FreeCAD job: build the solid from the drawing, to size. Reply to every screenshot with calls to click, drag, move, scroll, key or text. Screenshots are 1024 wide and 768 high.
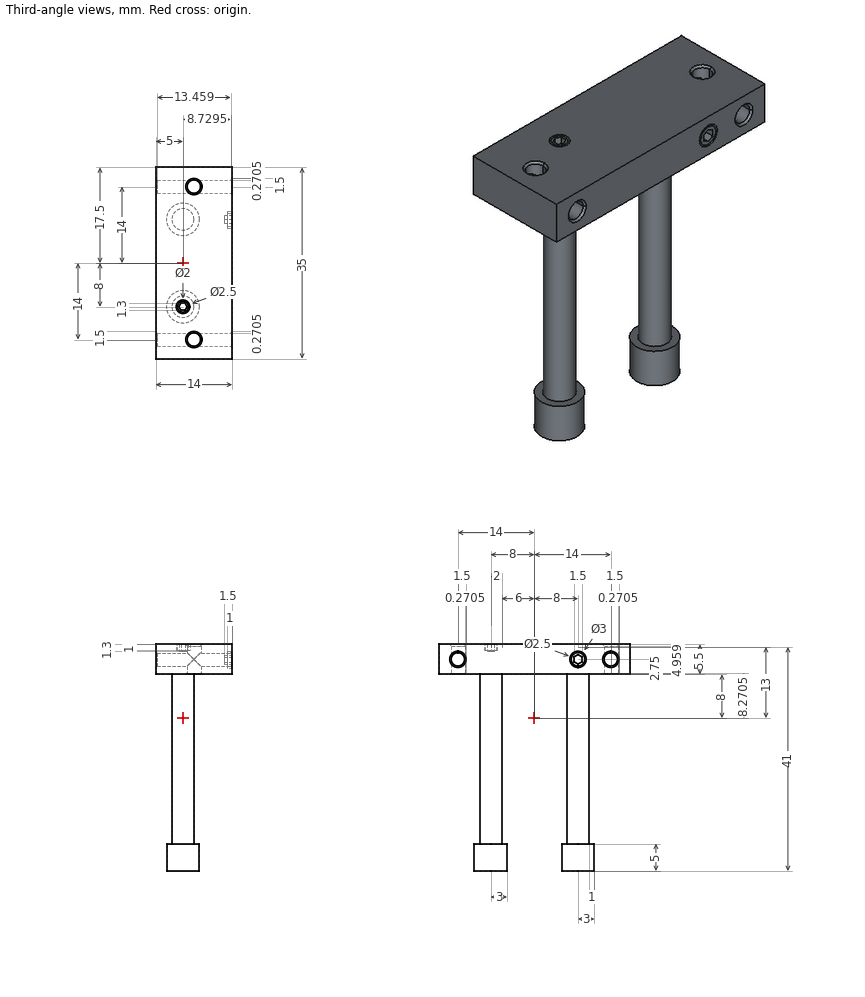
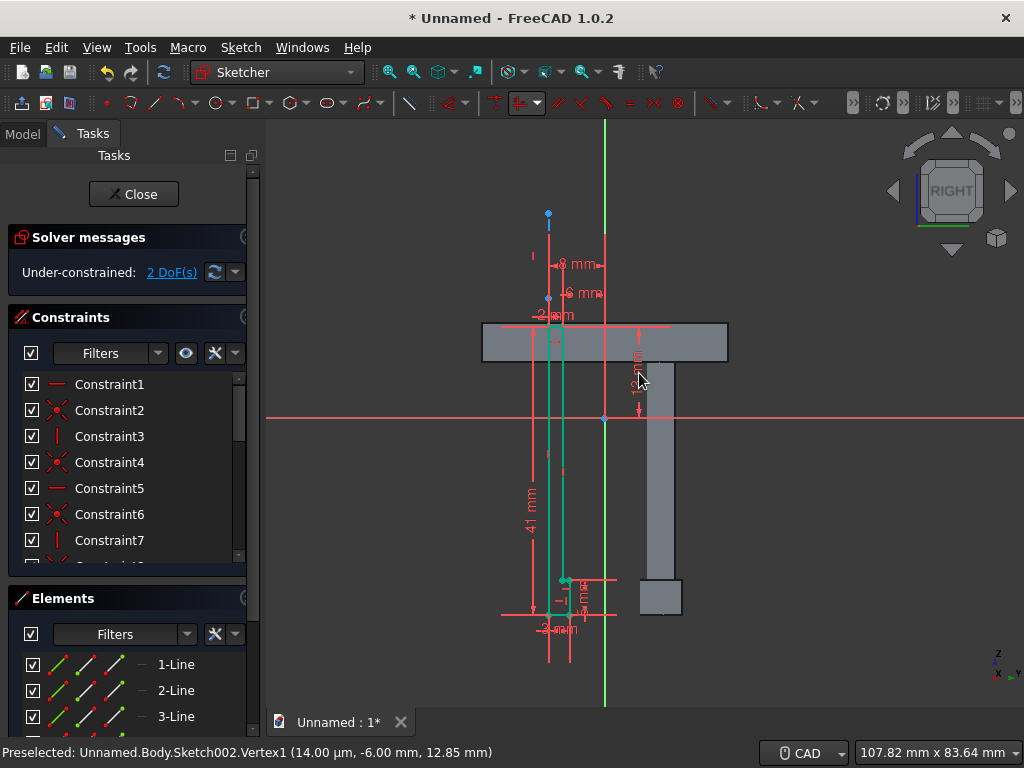
click(134, 194)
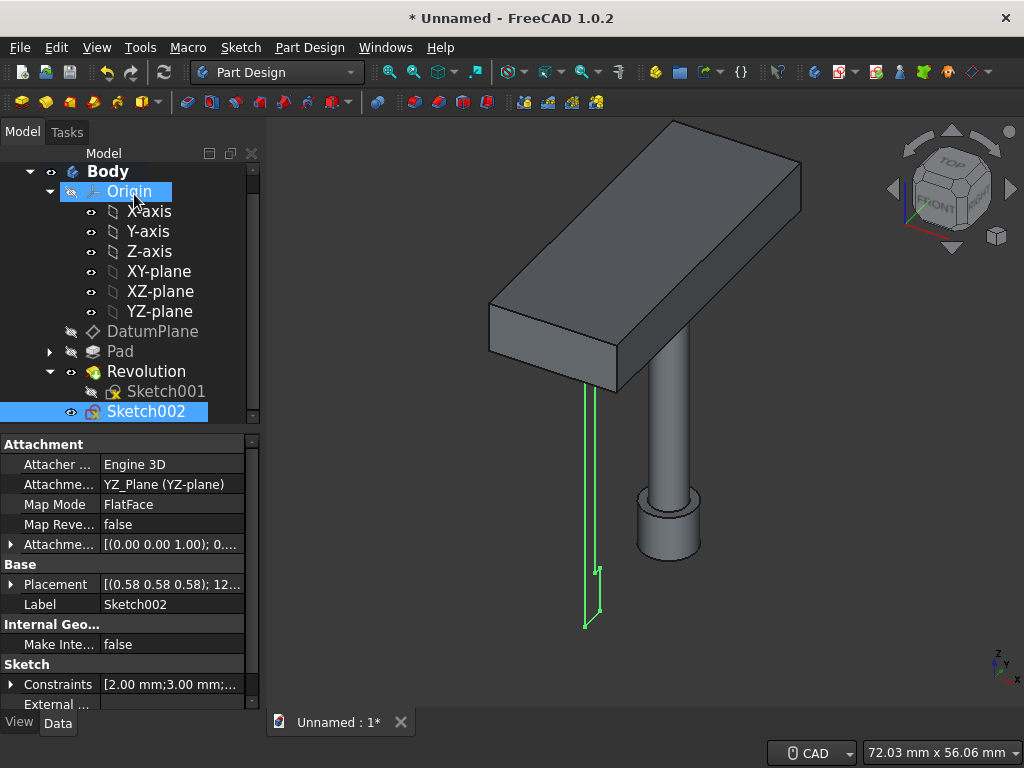
click(46, 102)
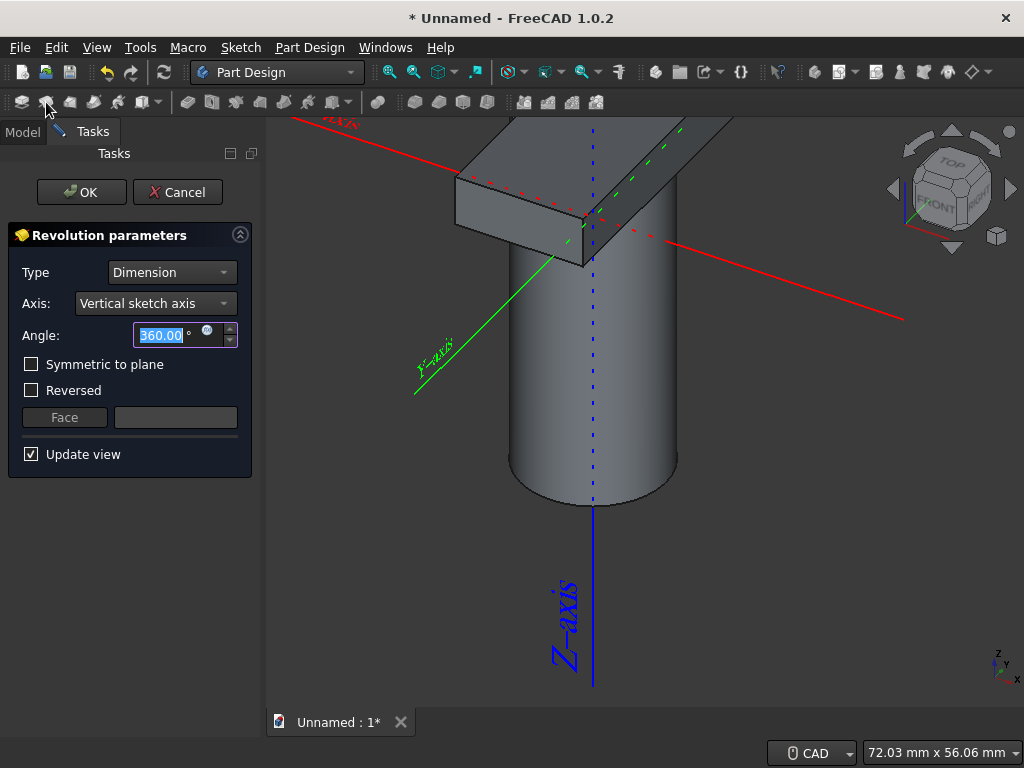
click(156, 304)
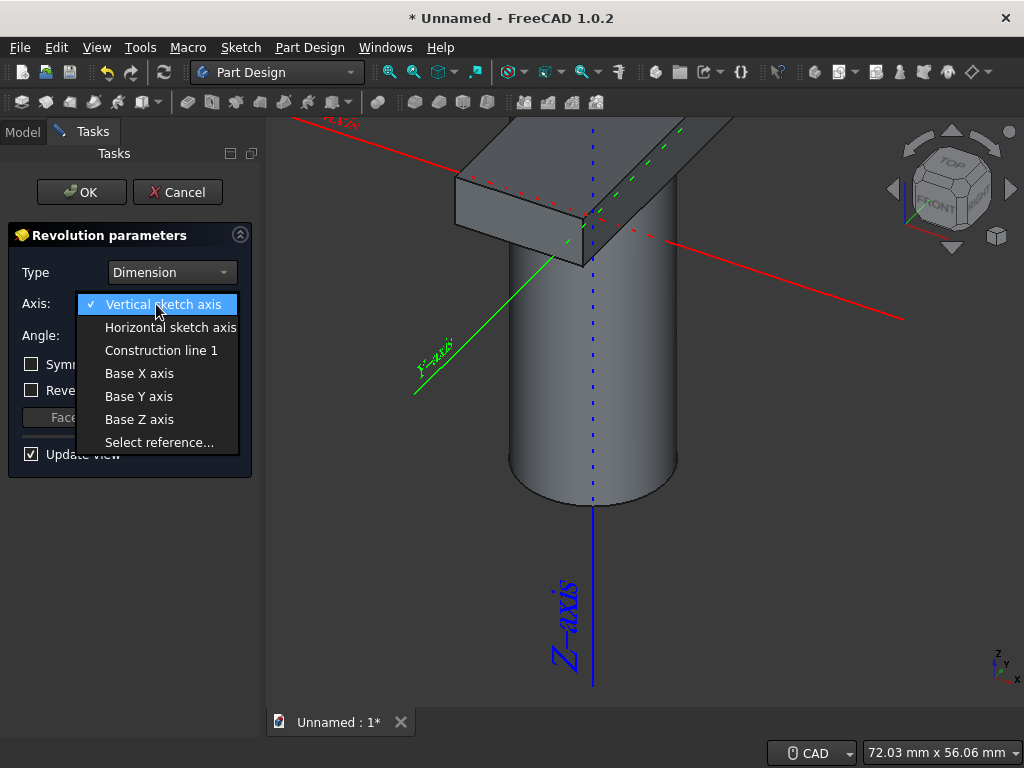
click(156, 350)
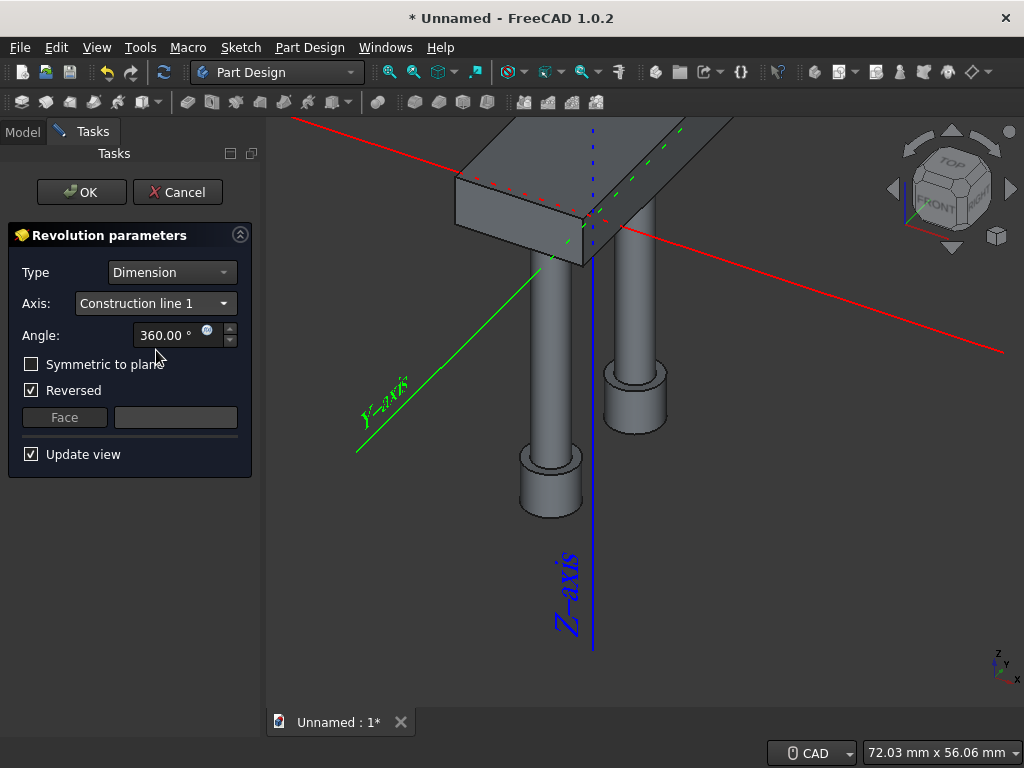
click(82, 192)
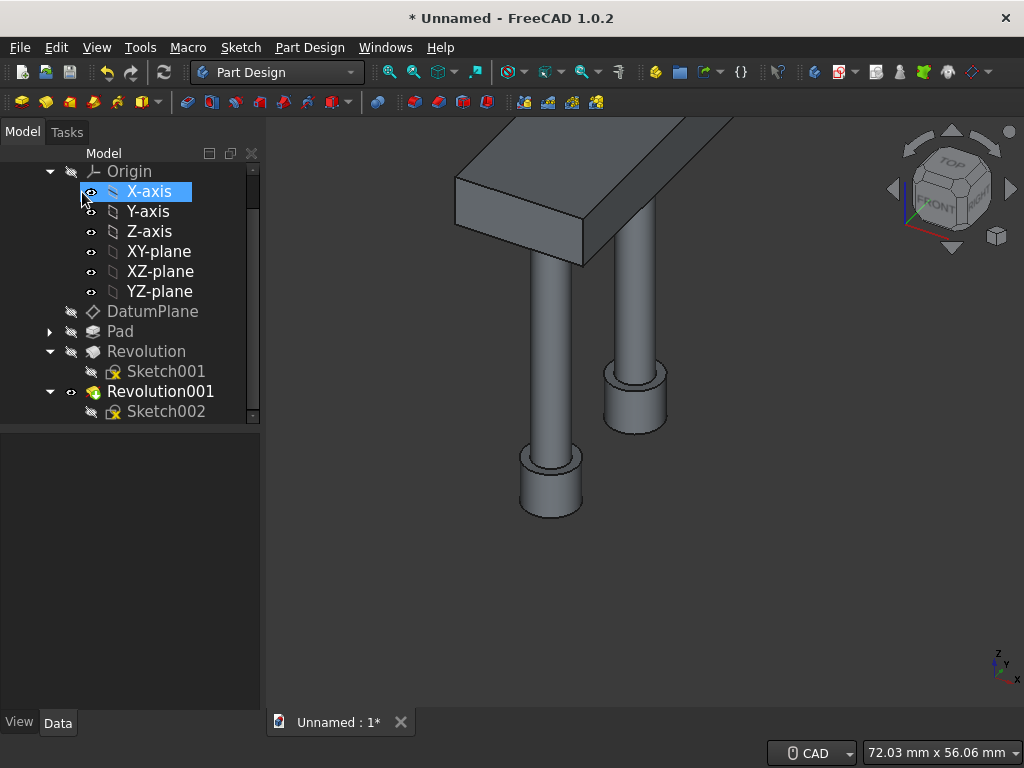
click(390, 72)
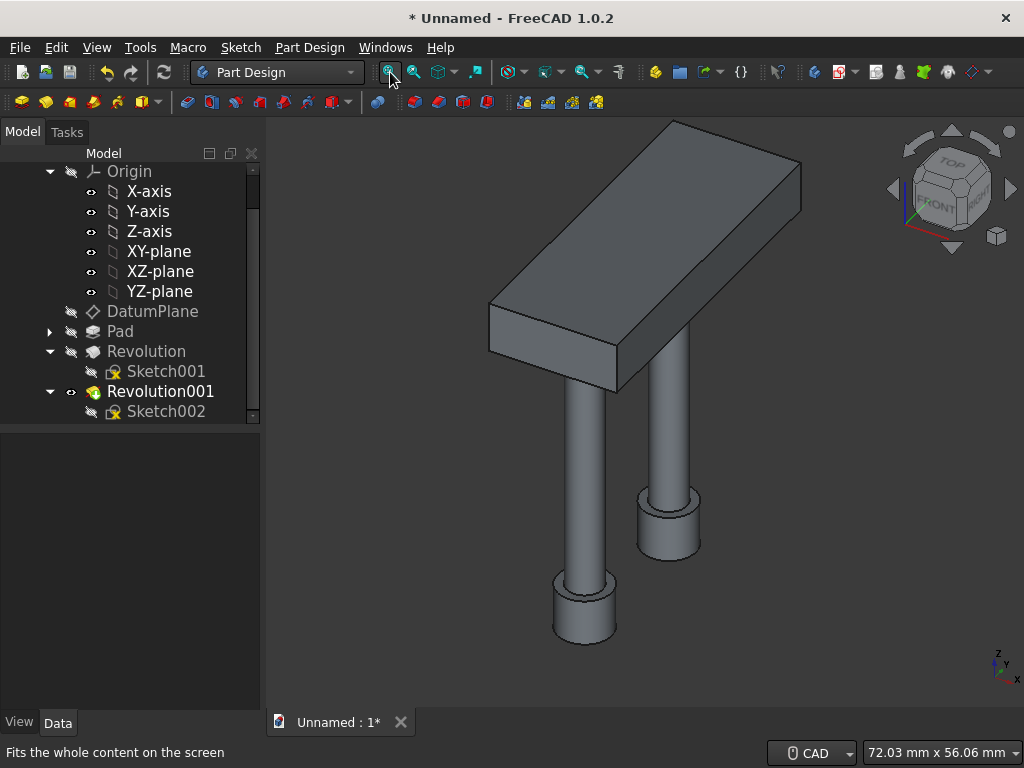
click(136, 292)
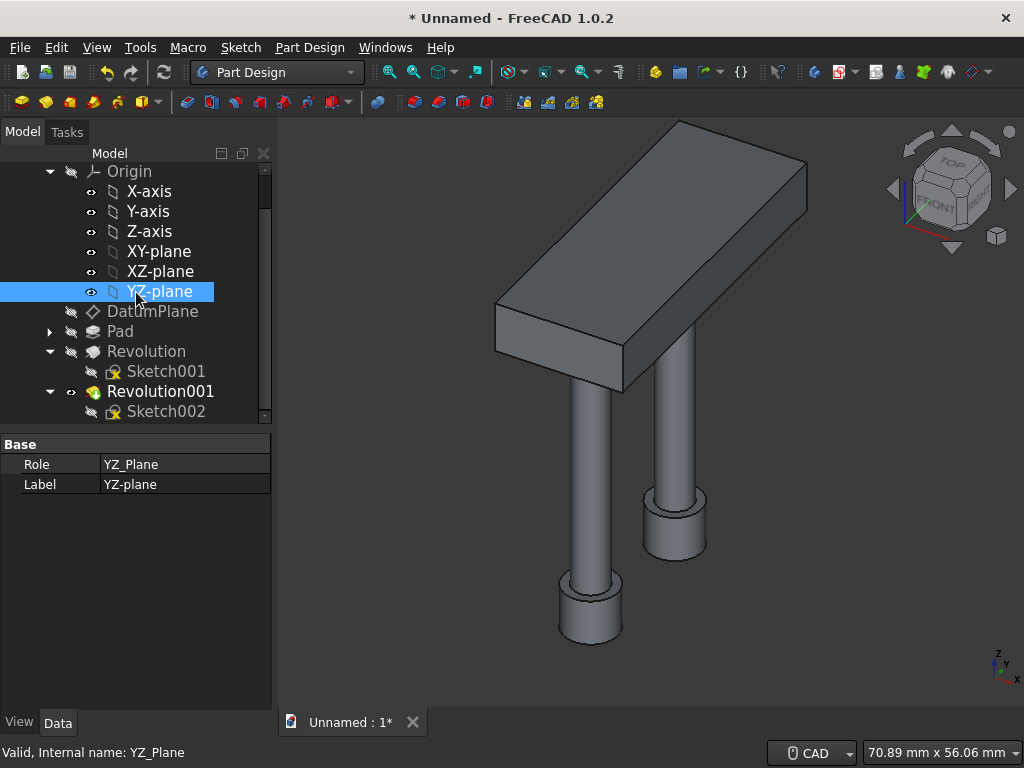
click(972, 72)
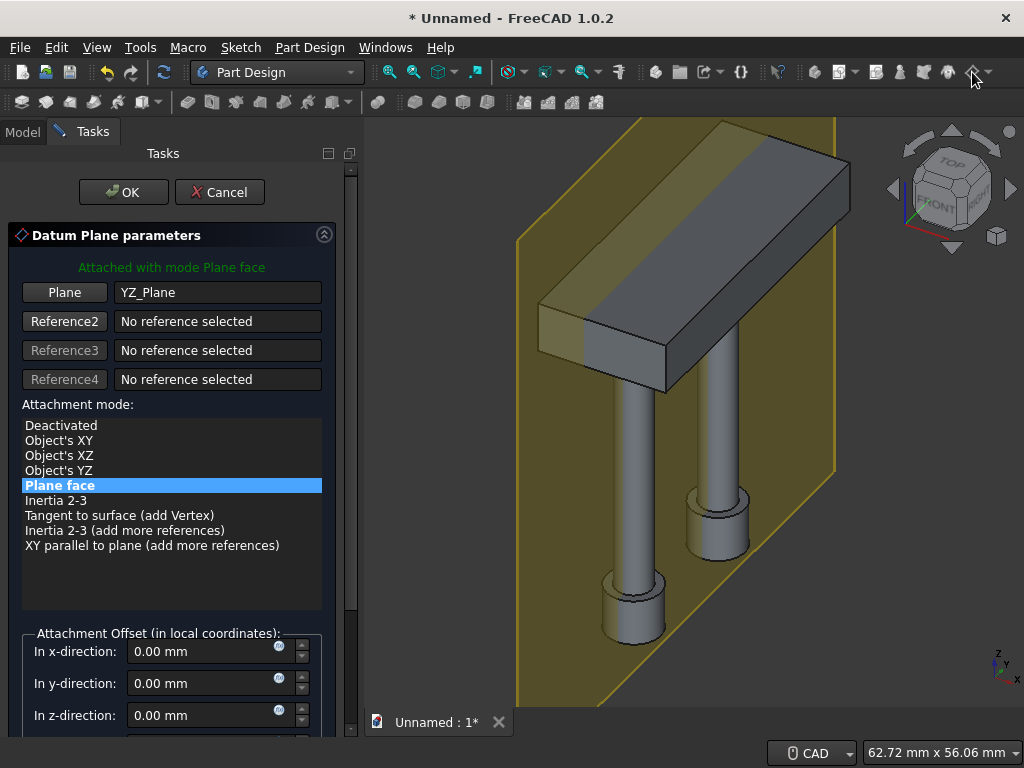
triple_click(210, 715)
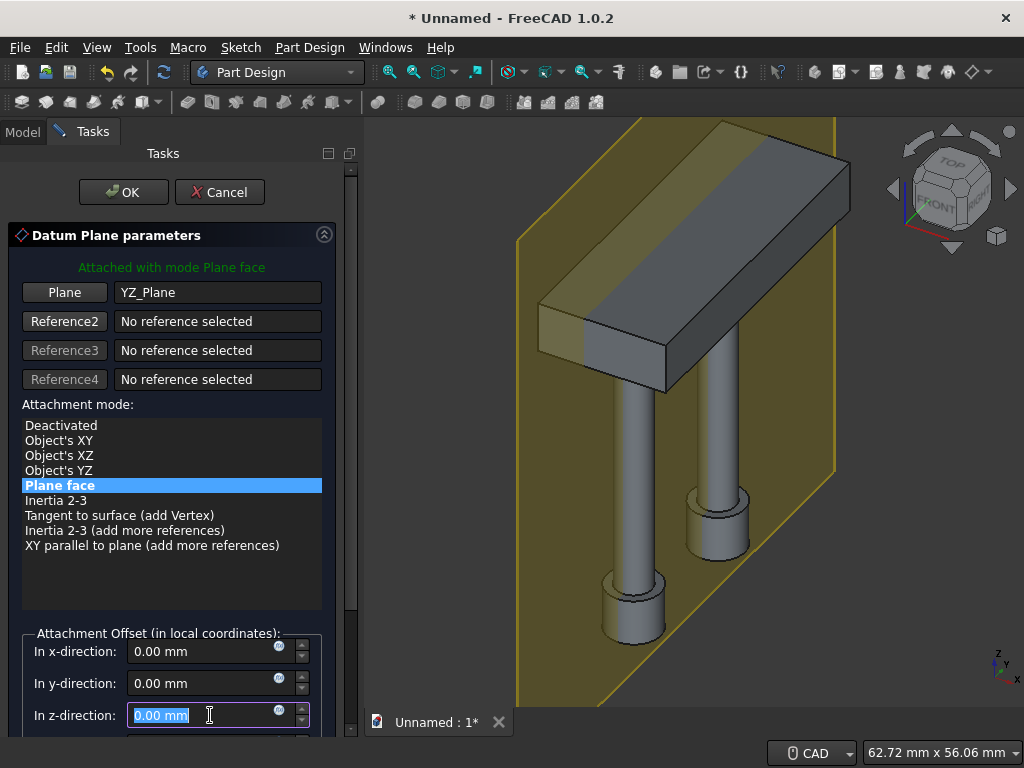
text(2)
key(Tab)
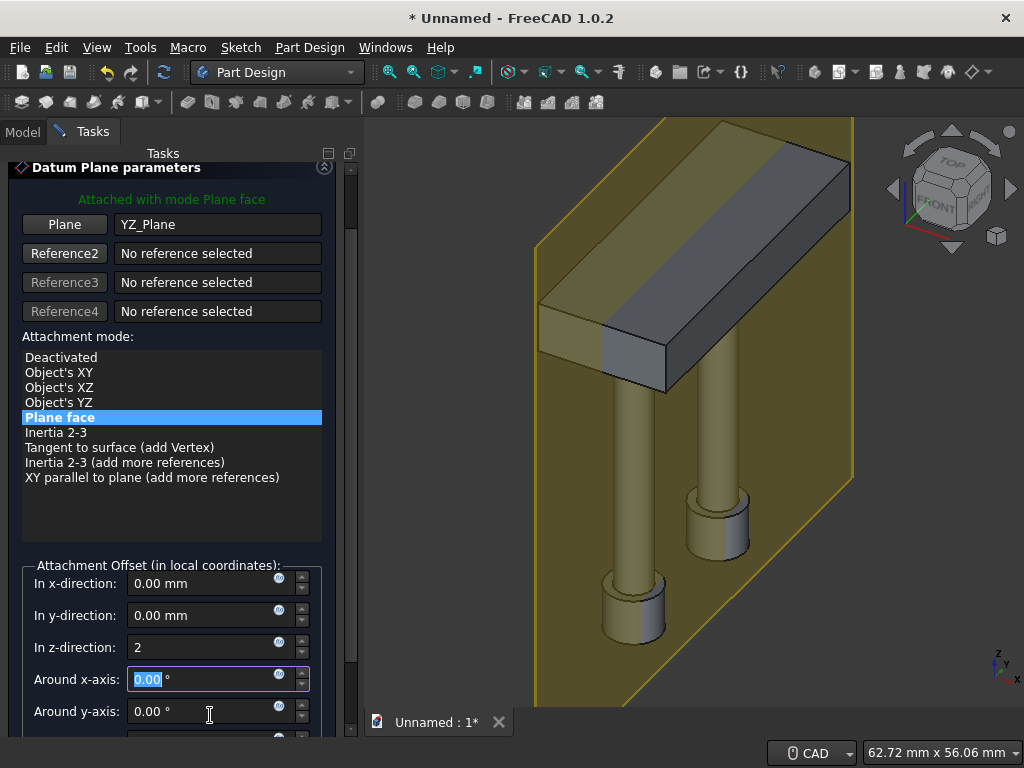
scroll(351, 450, up, 2)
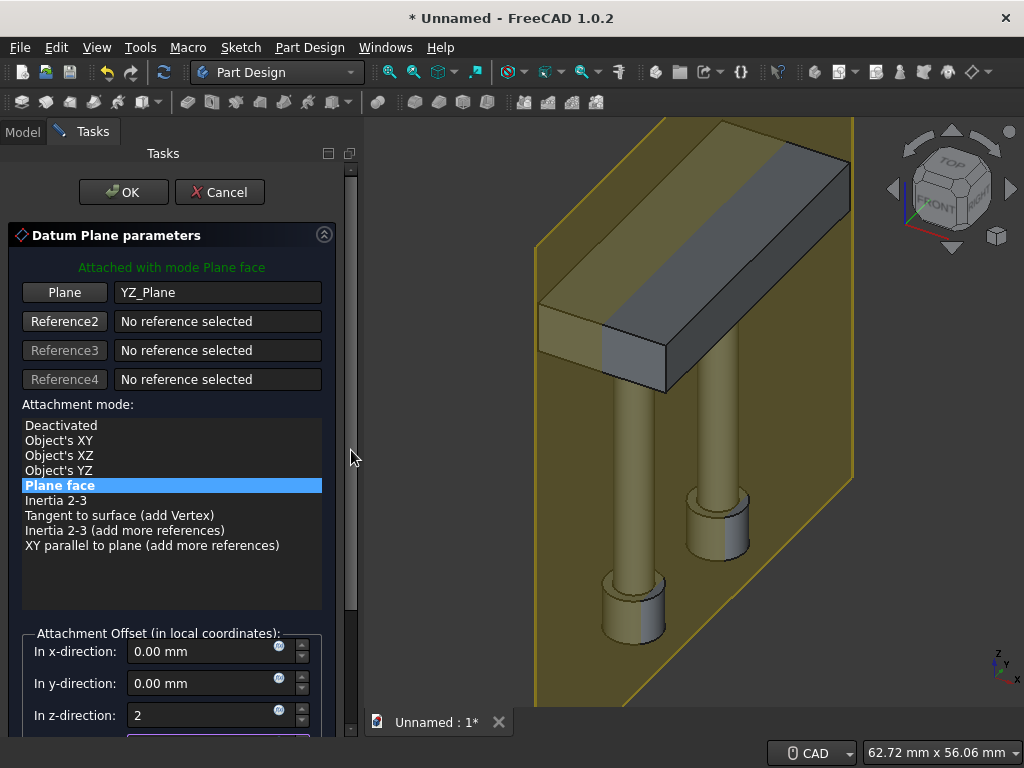
click(124, 192)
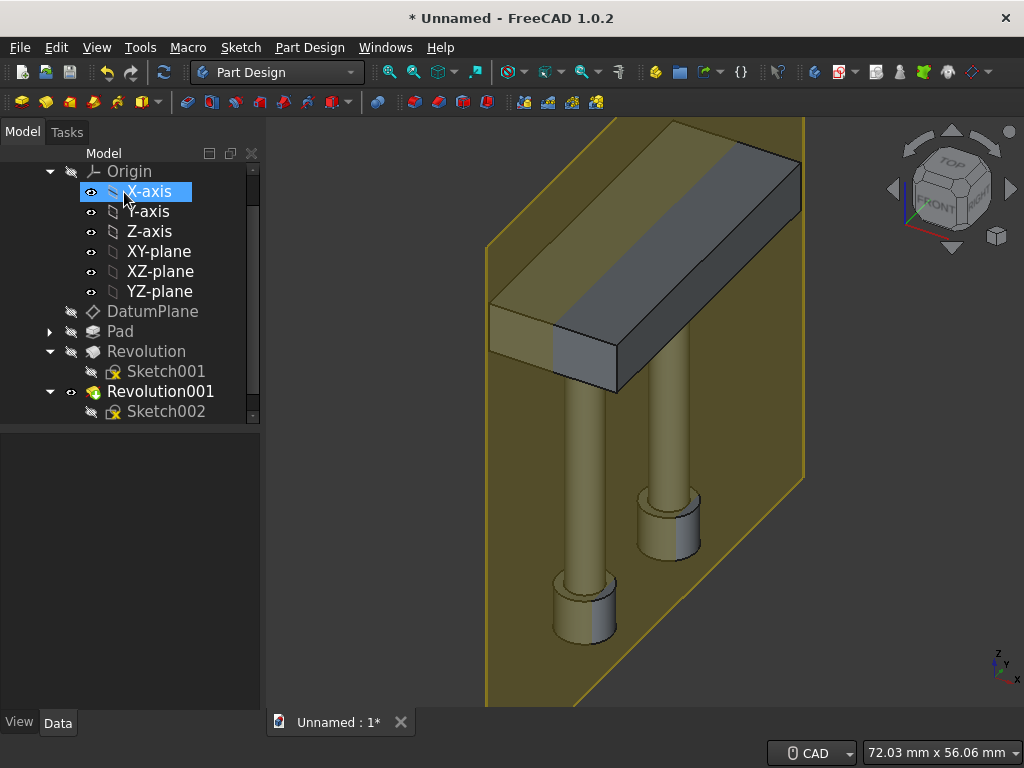
scroll(140, 287, down, 3)